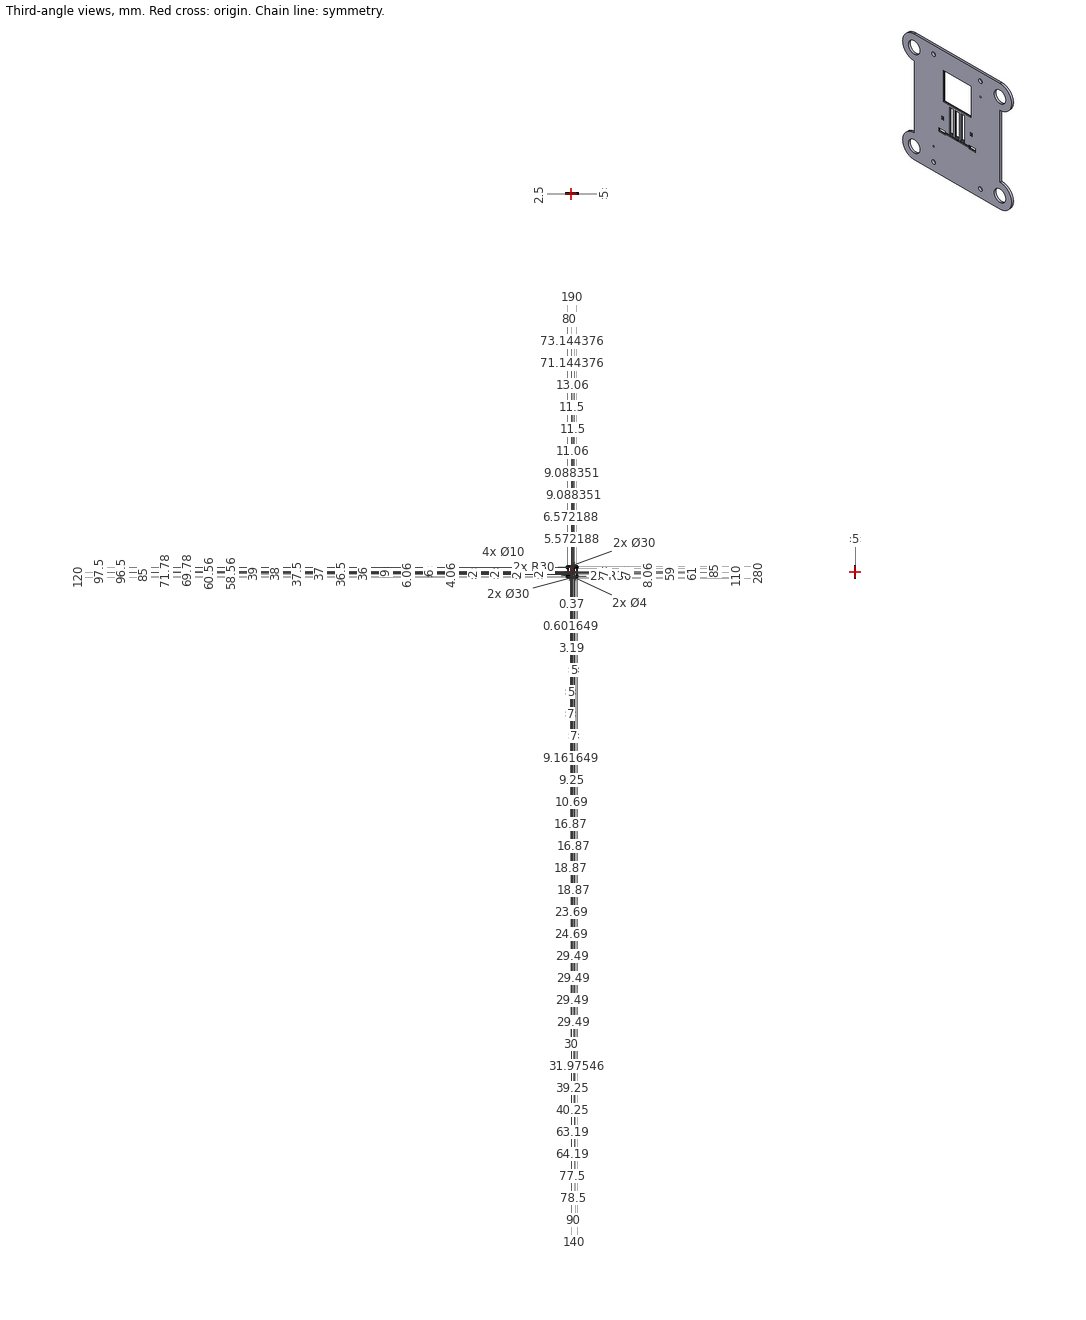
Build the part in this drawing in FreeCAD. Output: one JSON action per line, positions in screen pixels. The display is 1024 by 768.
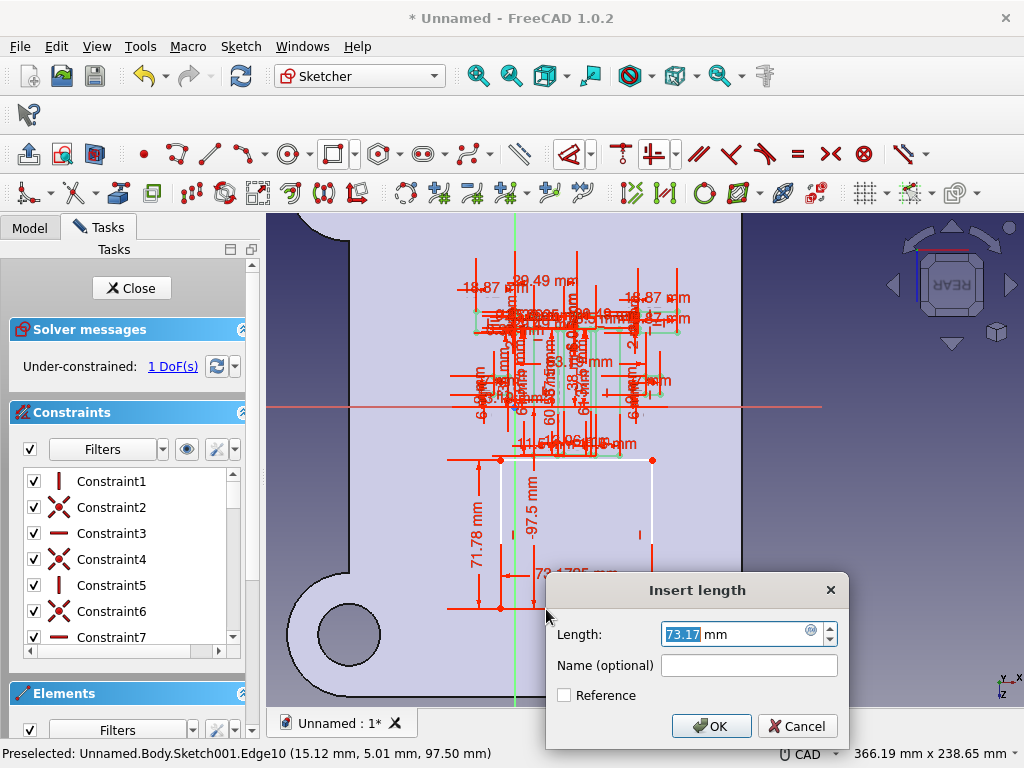
{"action": "type", "text": "73.144376"}
{"action": "key", "text": "Return"}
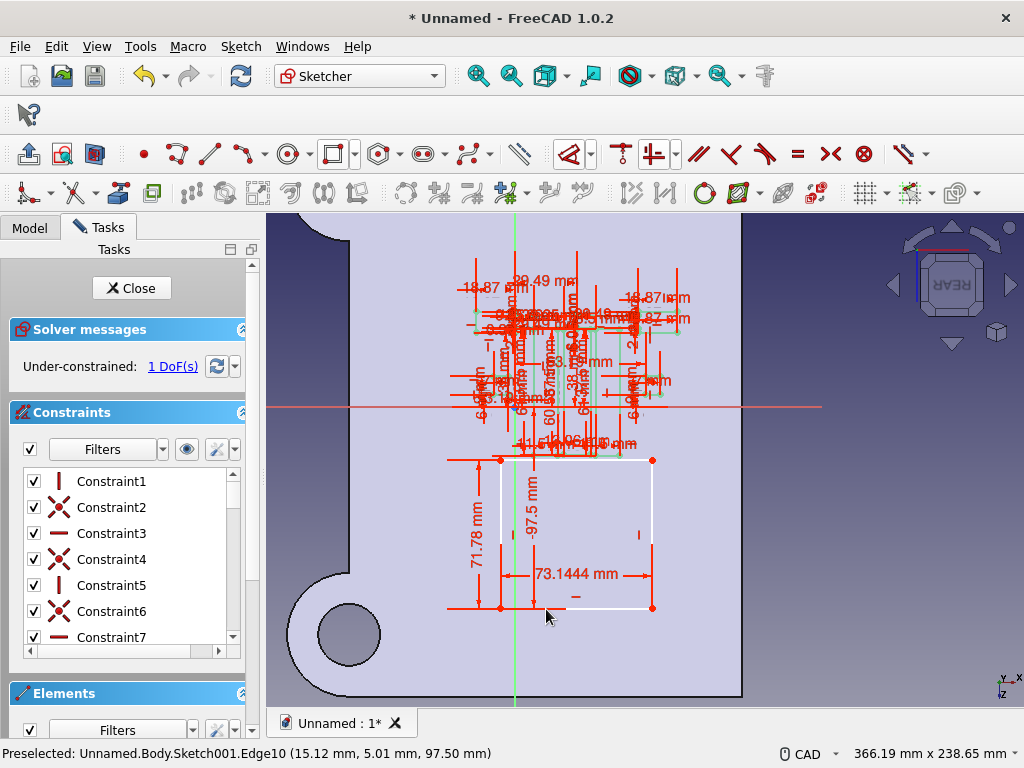
{"action": "scroll", "coordinate": [501, 460], "scroll_direction": "up", "scroll_amount": 6}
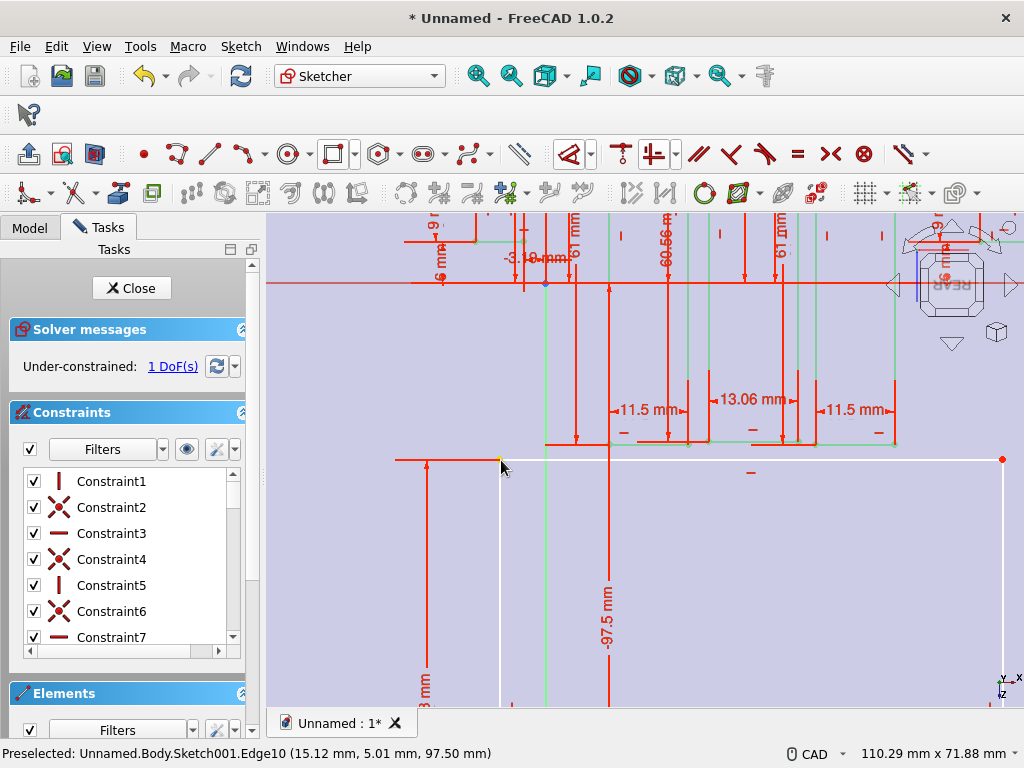
{"action": "left_click", "coordinate": [500, 460]}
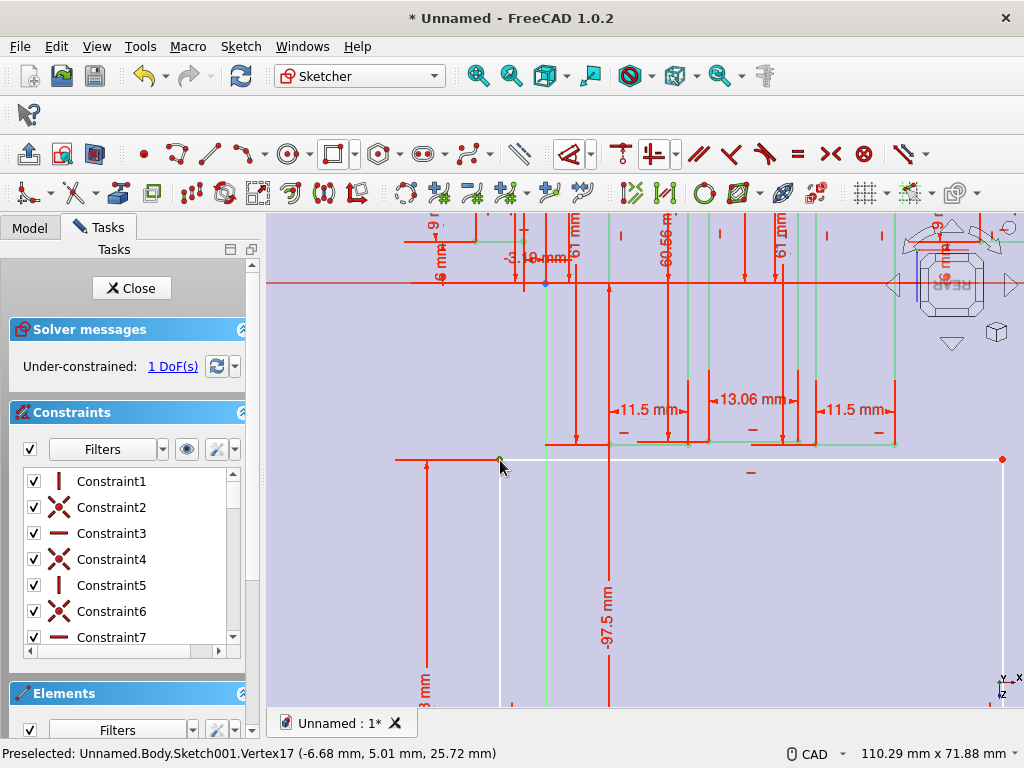
{"action": "key", "text": "l"}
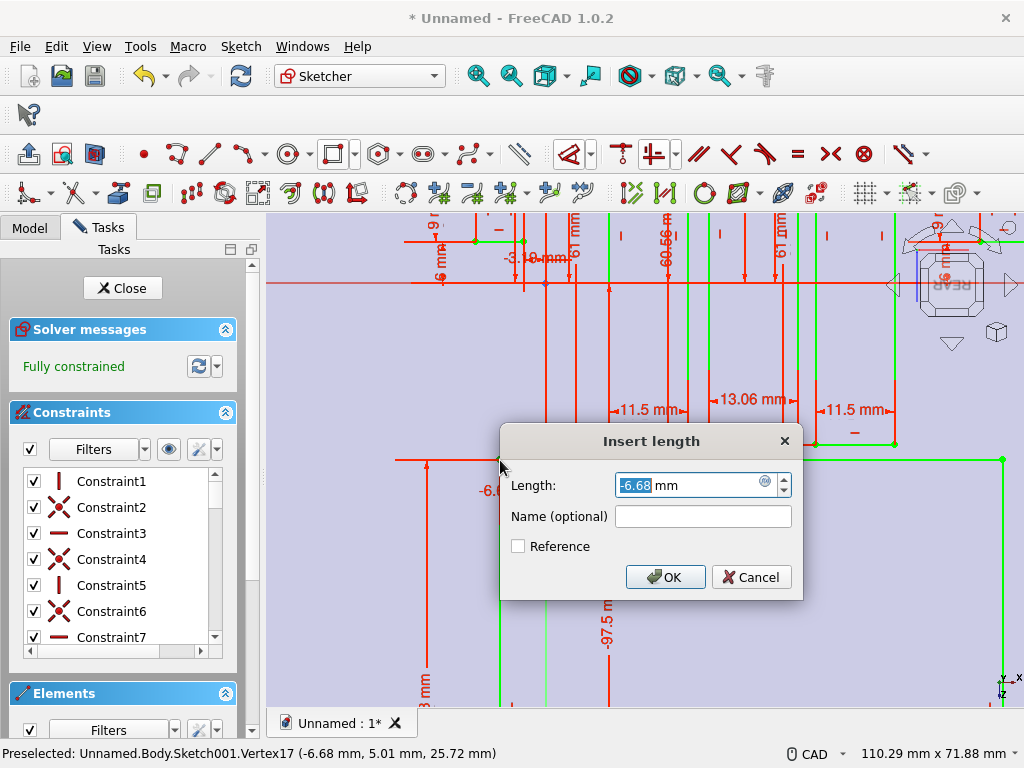
{"action": "type", "text": "-6.572188"}
{"action": "key", "text": "Return"}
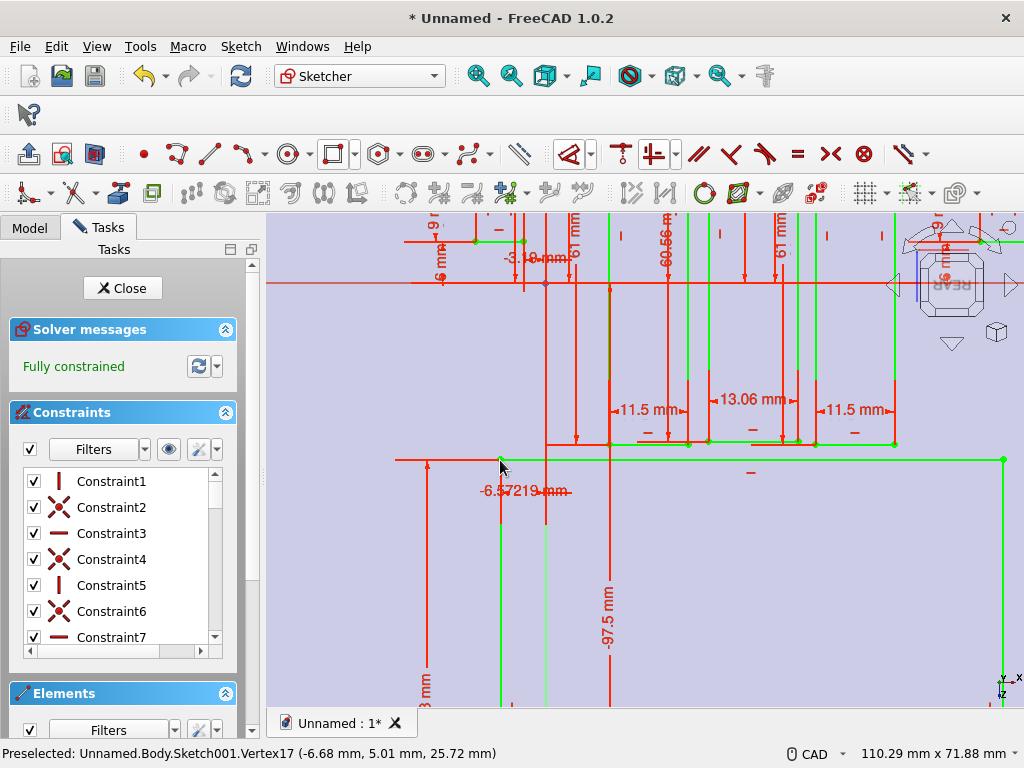
{"action": "left_click", "coordinate": [123, 288]}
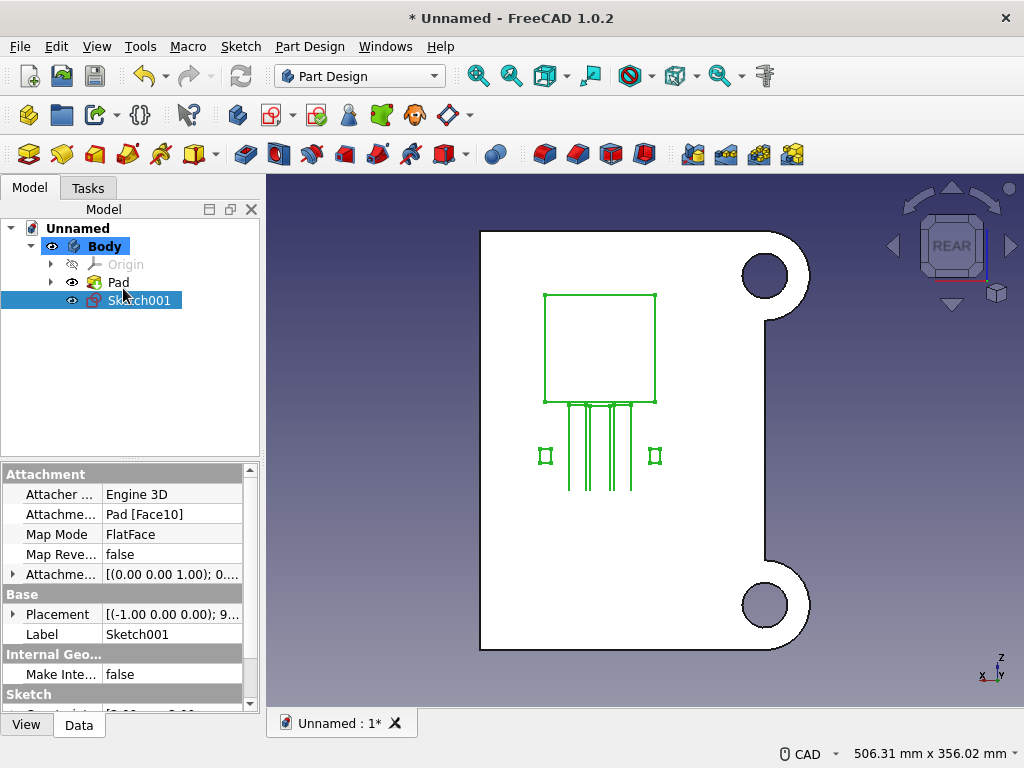
{"action": "left_click", "coordinate": [246, 154]}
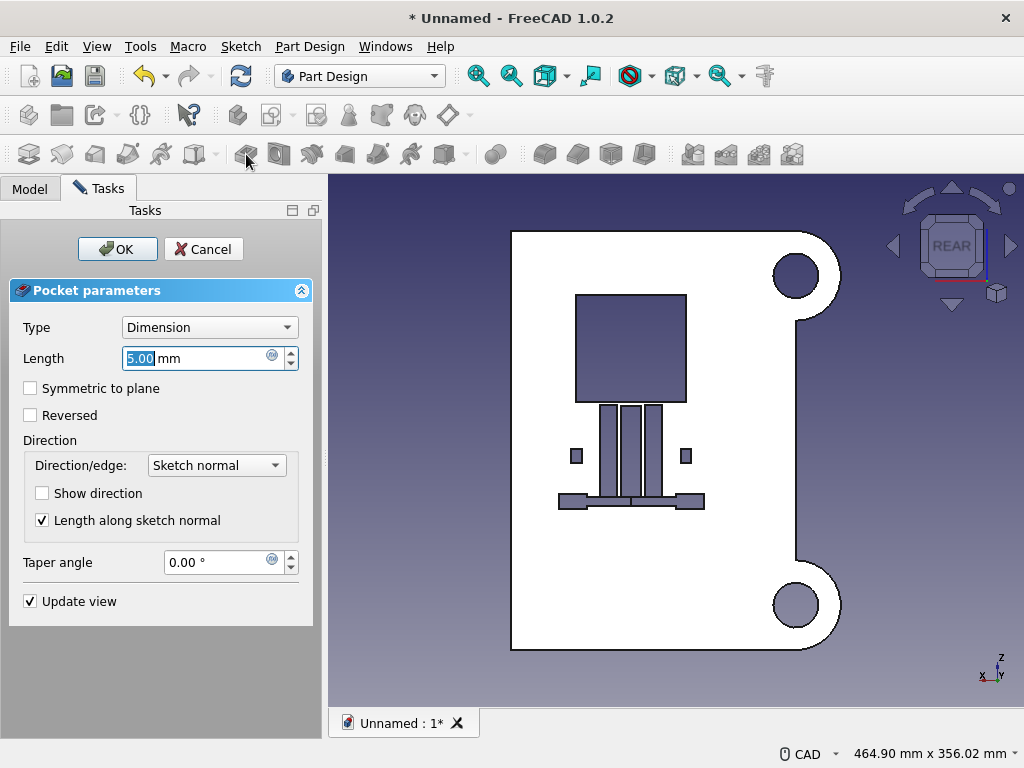
{"action": "type", "text": "2.5"}
{"action": "key", "text": "Tab"}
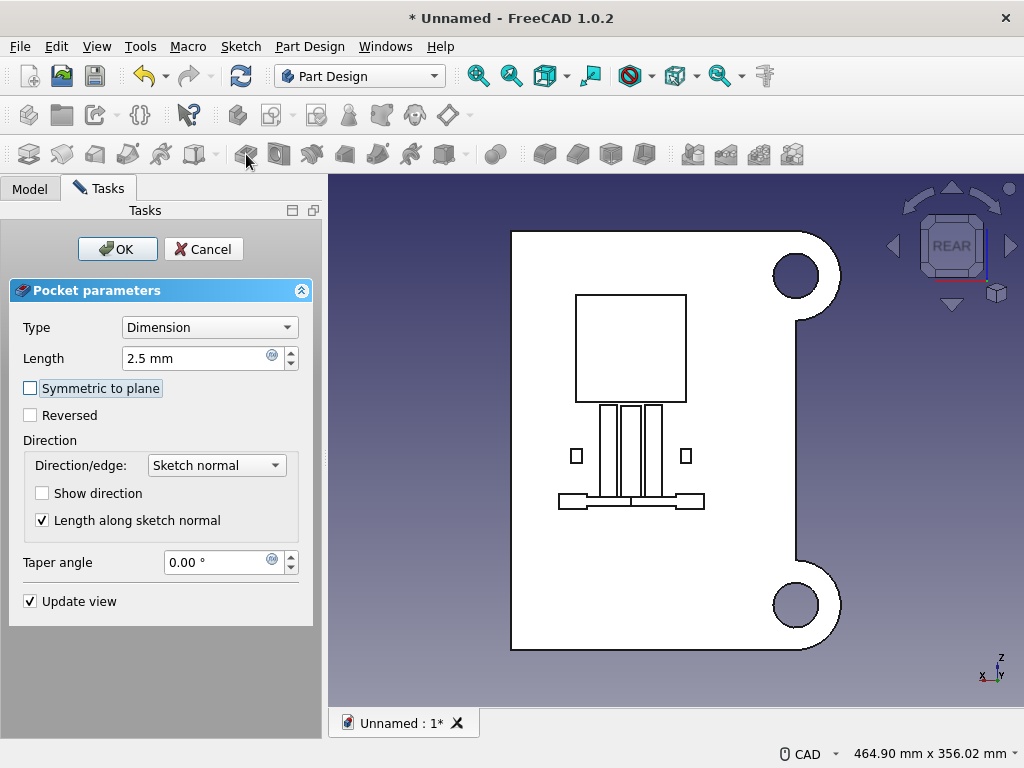
{"action": "left_click", "coordinate": [118, 249]}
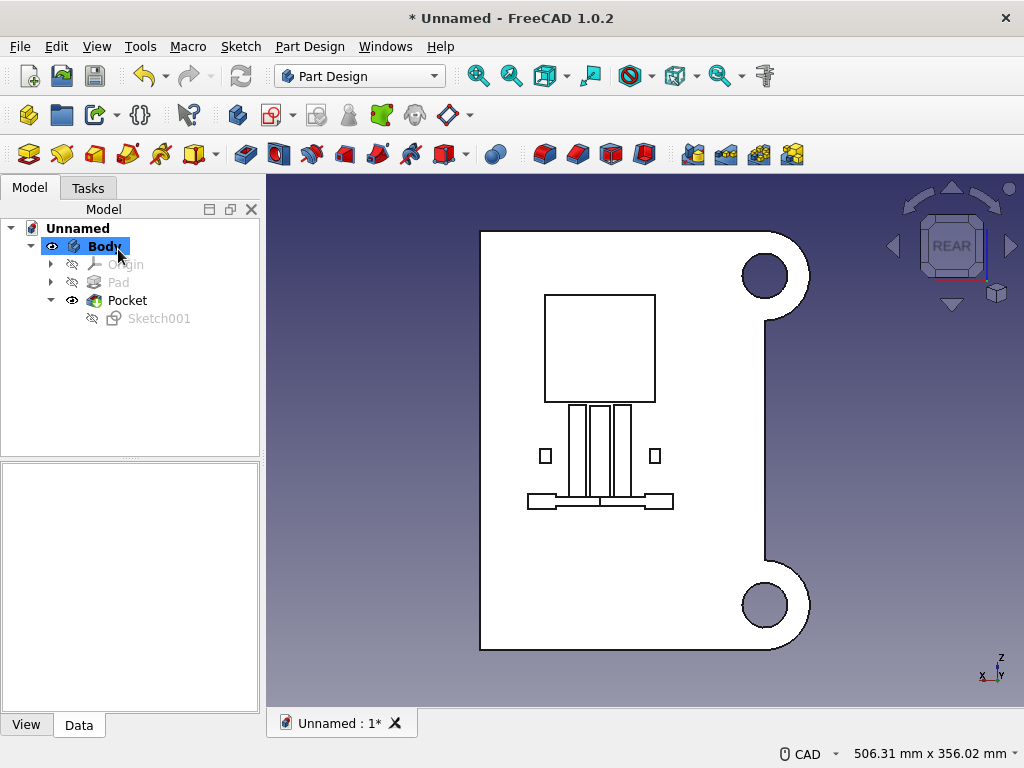
{"action": "left_click", "coordinate": [692, 559]}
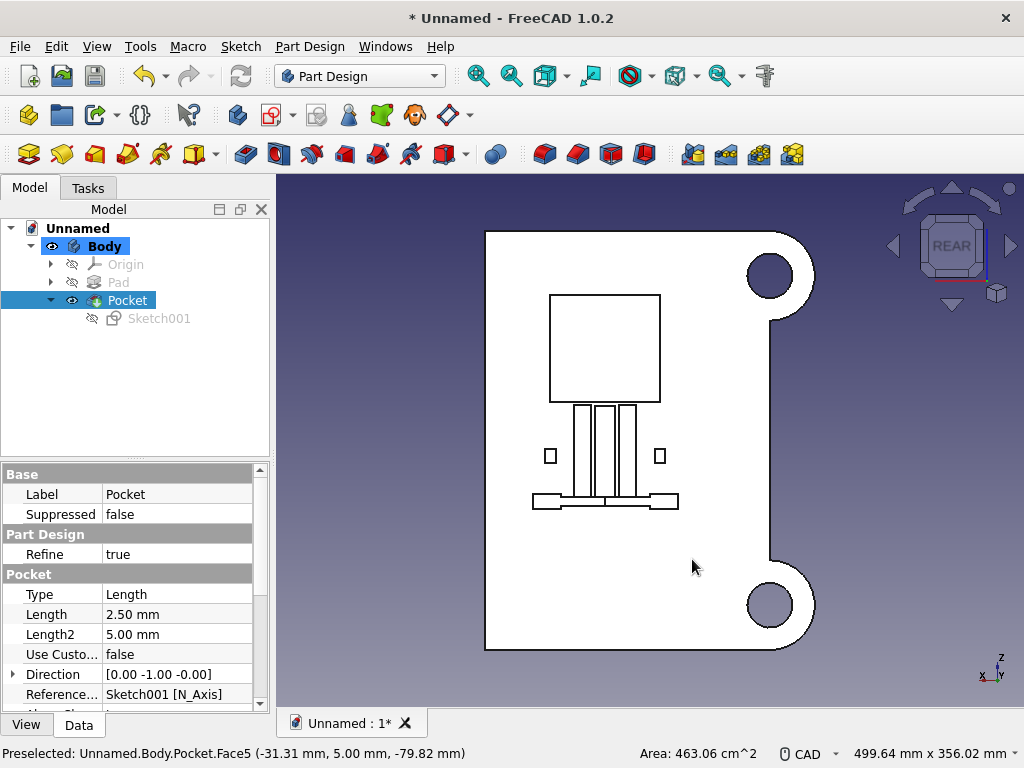
{"action": "left_click", "coordinate": [270, 116]}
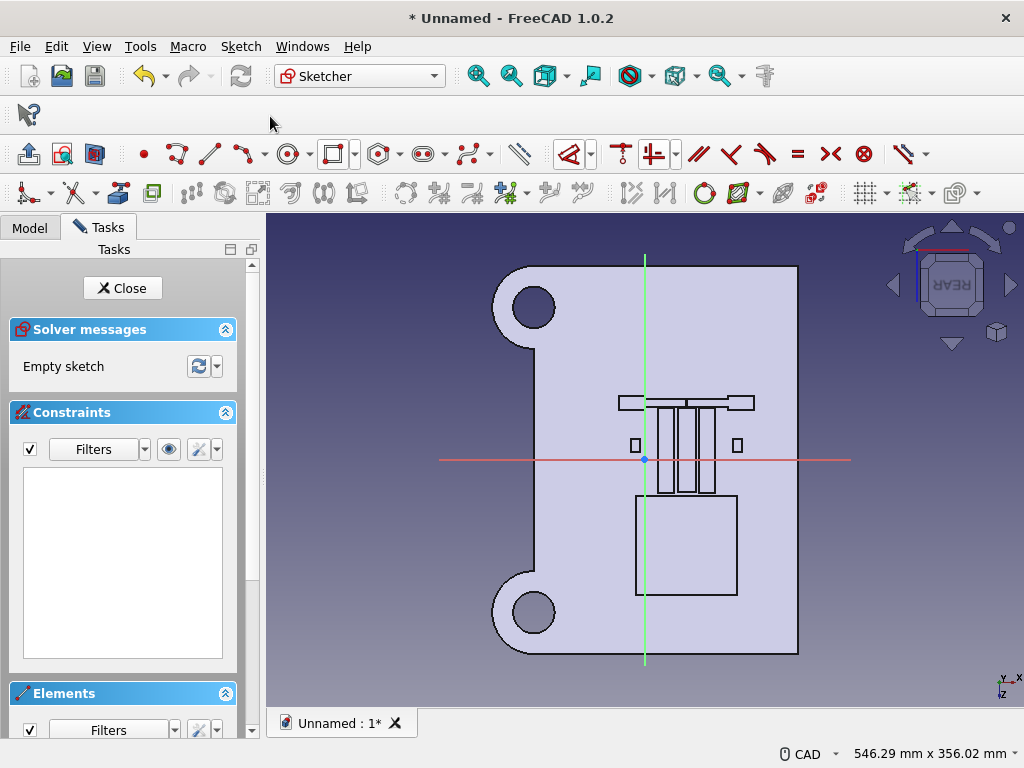
{"action": "scroll", "coordinate": [859, 568], "scroll_direction": "up", "scroll_amount": 2}